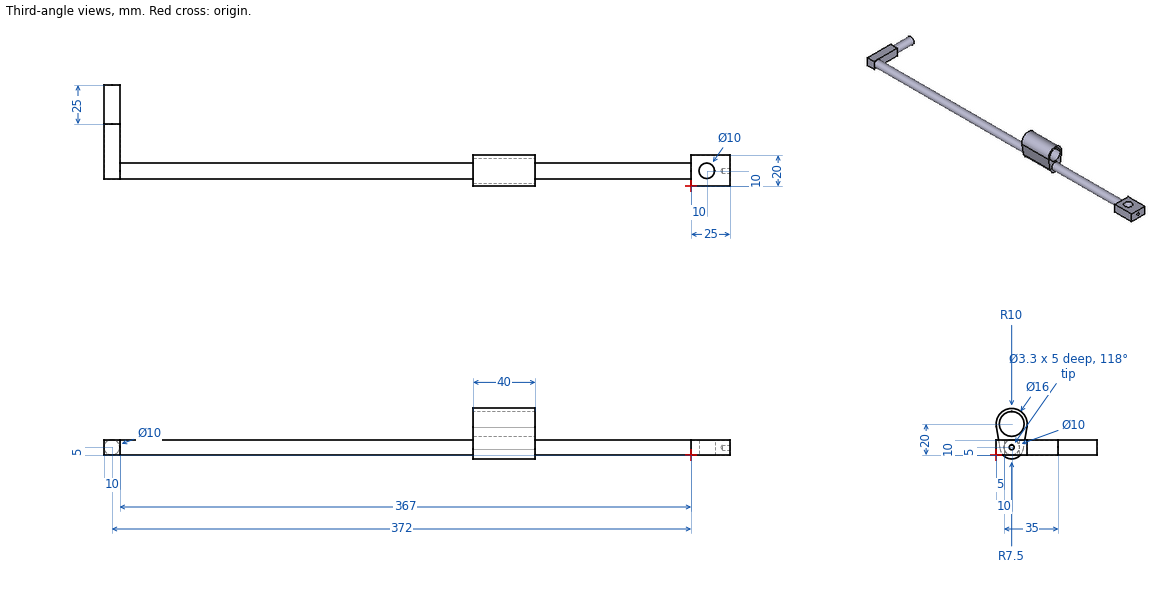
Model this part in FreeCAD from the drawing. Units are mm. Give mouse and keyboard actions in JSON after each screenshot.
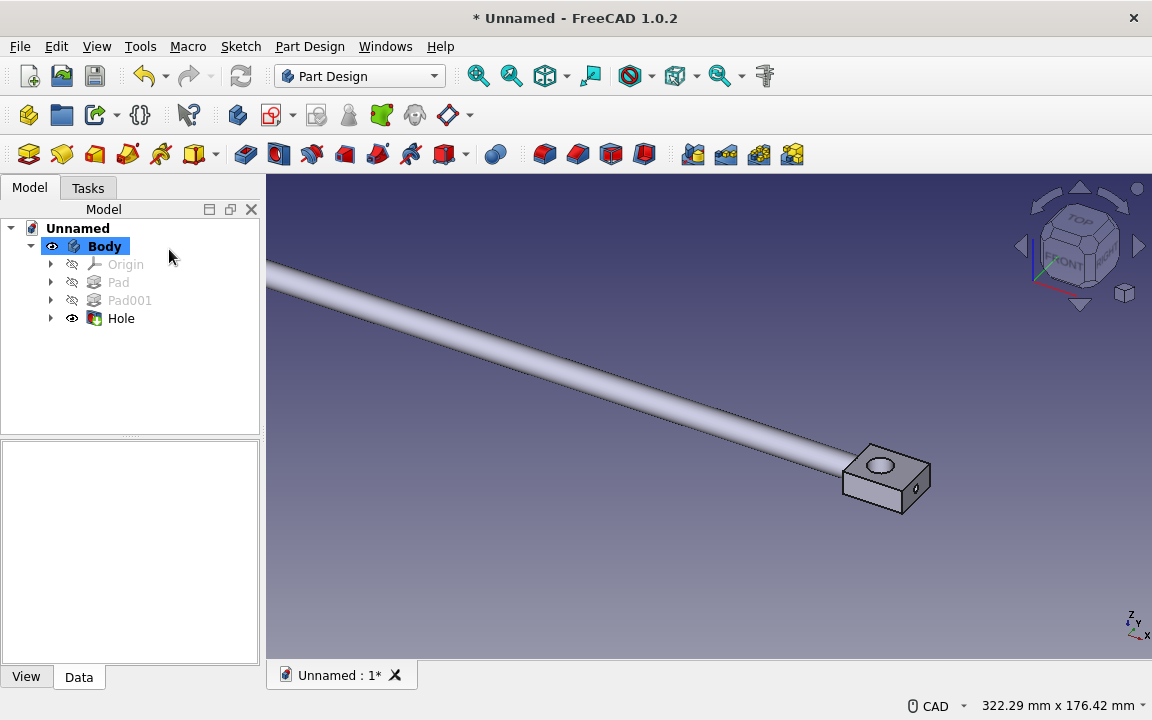
{"action": "key", "text": "v f"}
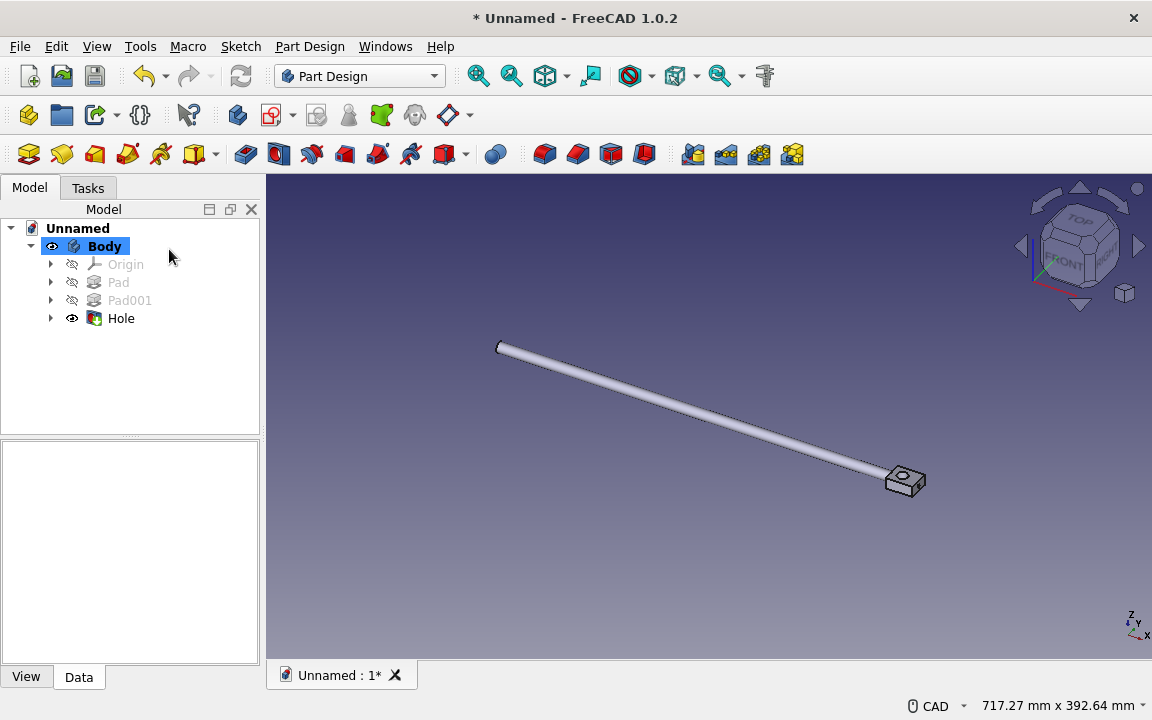
{"action": "key", "text": "6"}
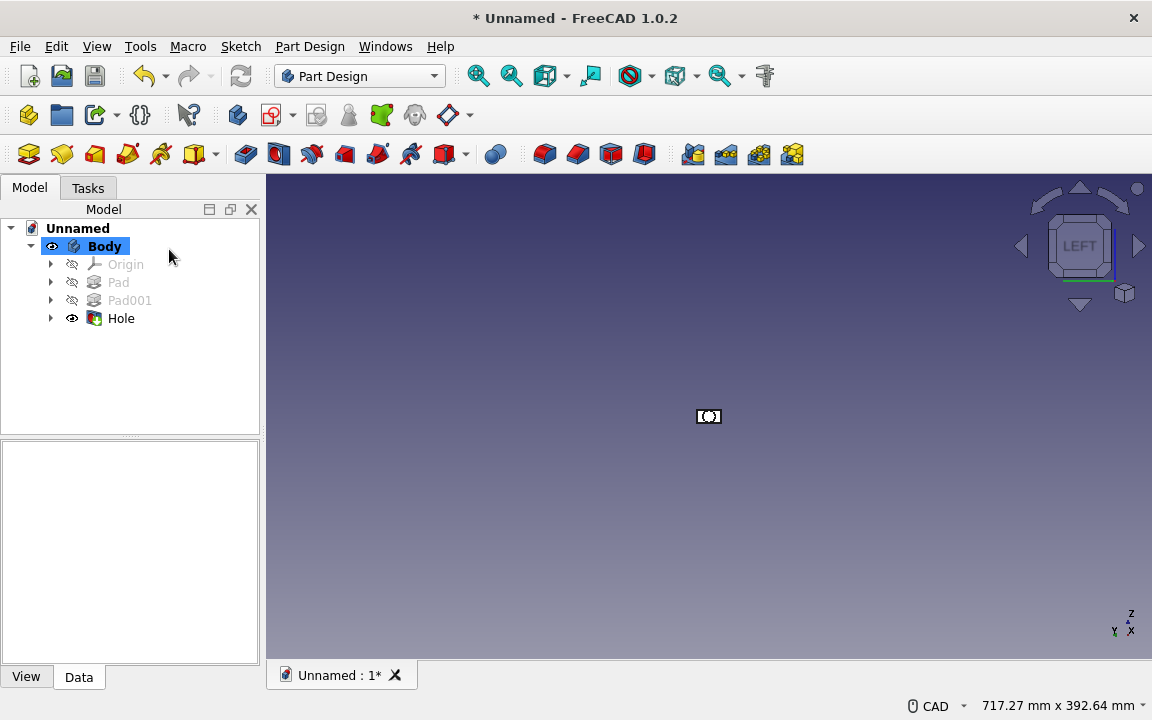
{"action": "left_click", "coordinate": [479, 76]}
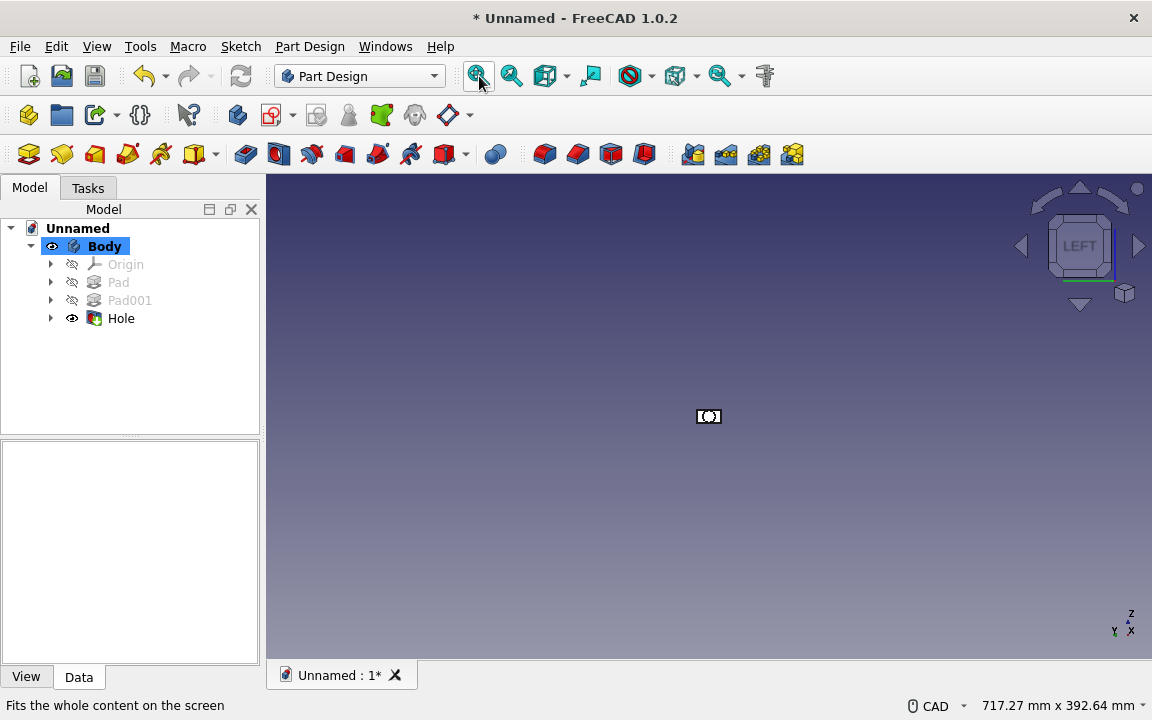
{"action": "scroll", "coordinate": [709, 415], "scroll_direction": "up", "scroll_amount": 4}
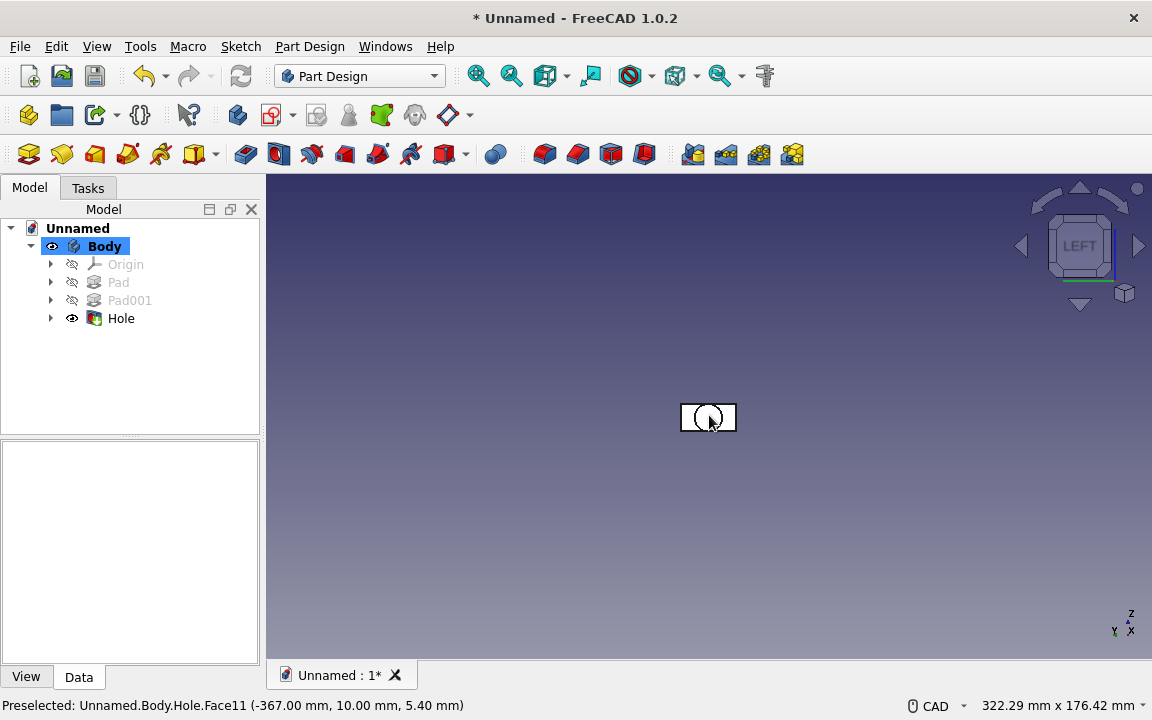
{"action": "left_click", "coordinate": [708, 417]}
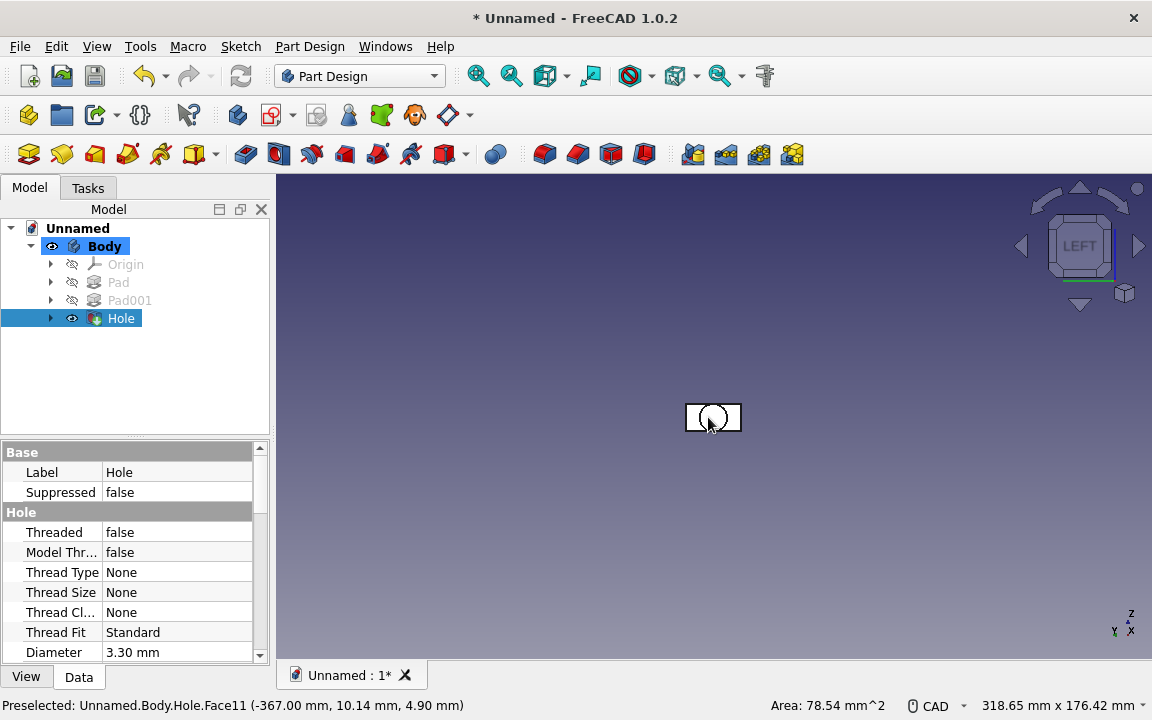
{"action": "left_click", "coordinate": [270, 116]}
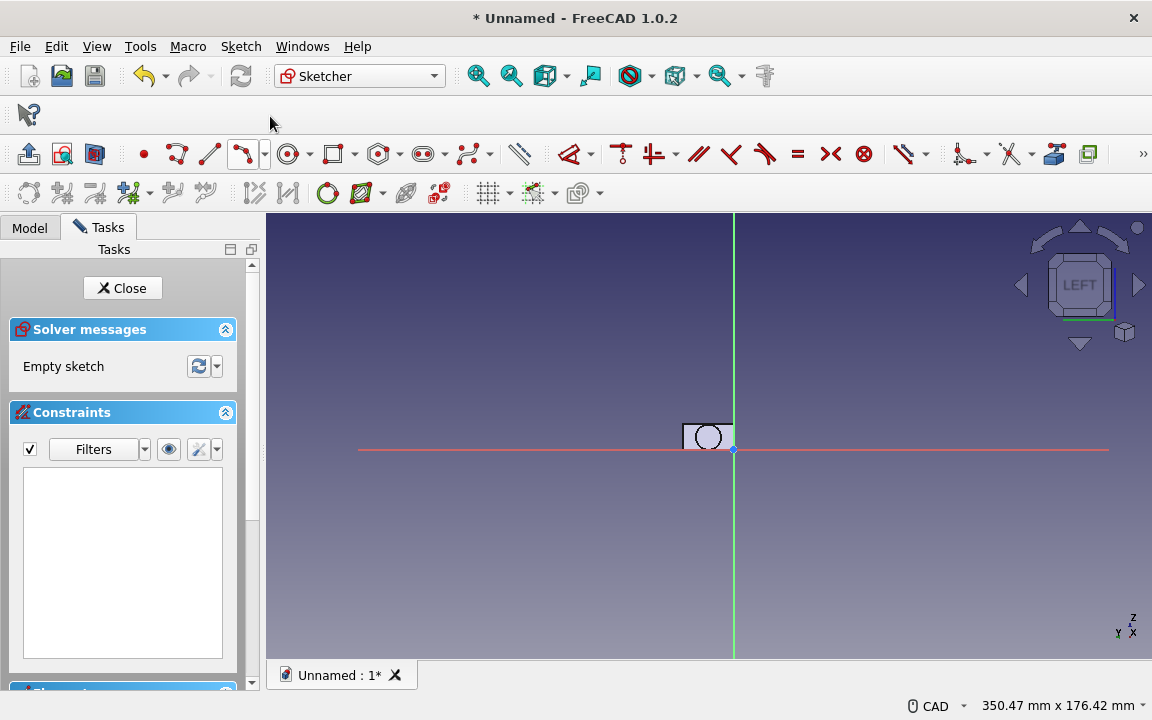
{"action": "scroll", "coordinate": [694, 437], "scroll_direction": "up", "scroll_amount": 8}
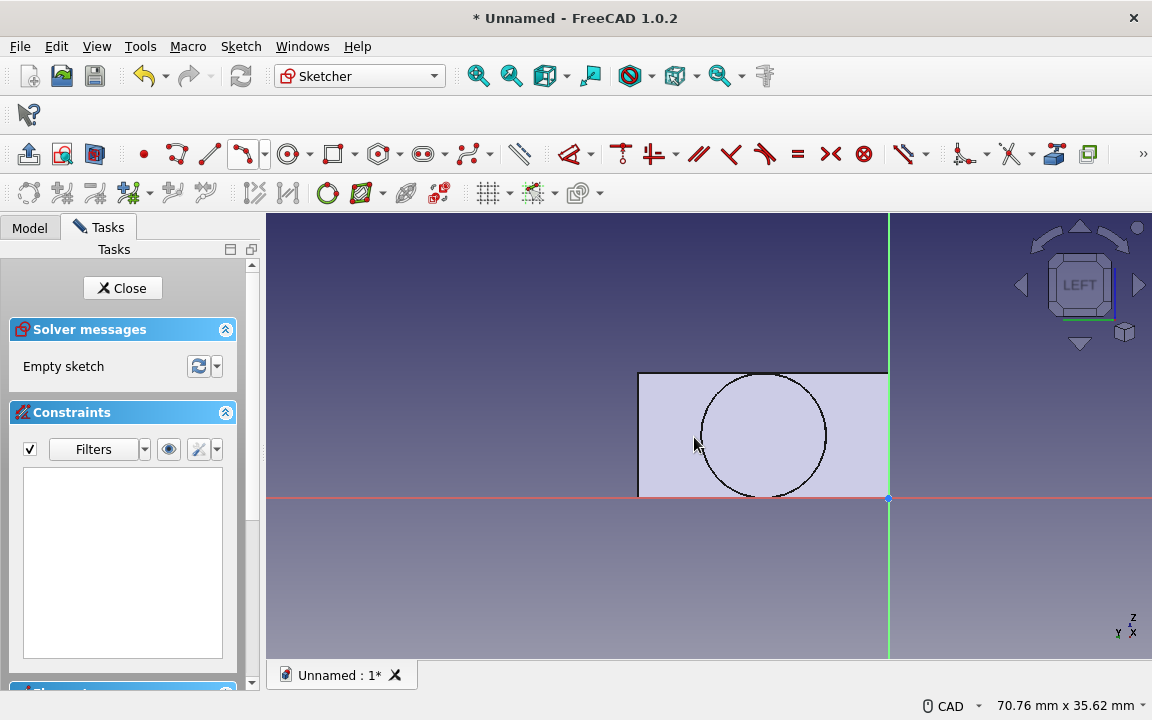
{"action": "key", "text": "g r"}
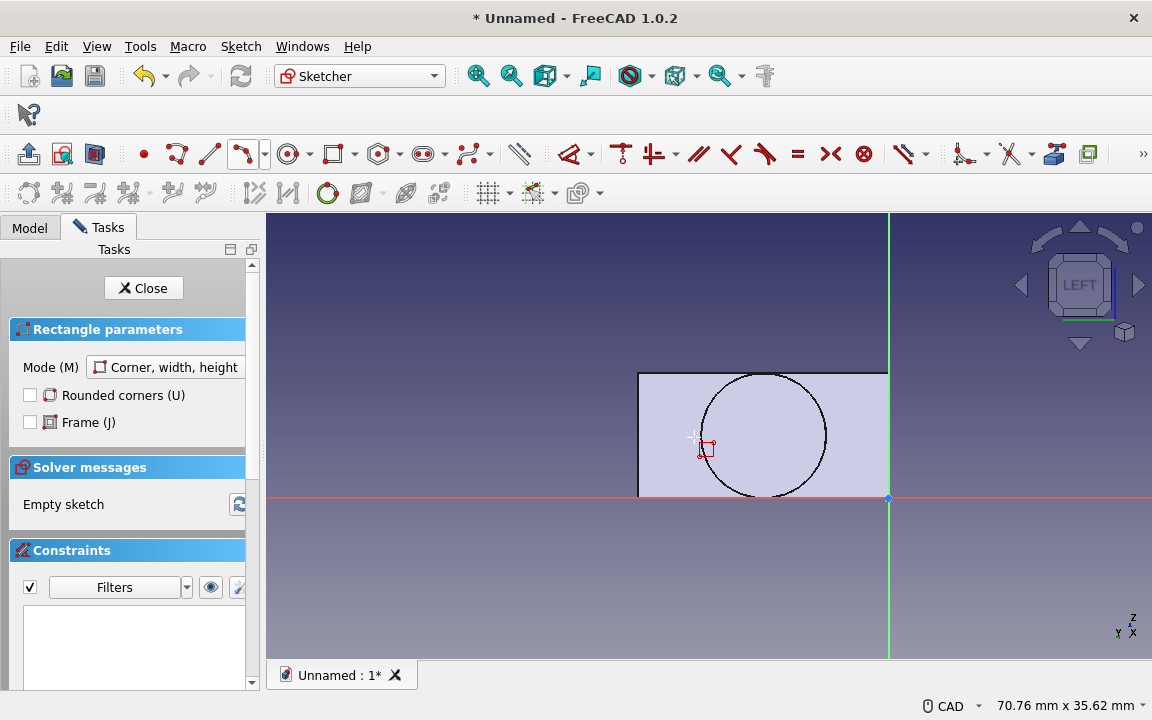
{"action": "left_click", "coordinate": [388, 373]}
{"action": "left_click", "coordinate": [826, 498]}
{"action": "key", "text": "Escape"}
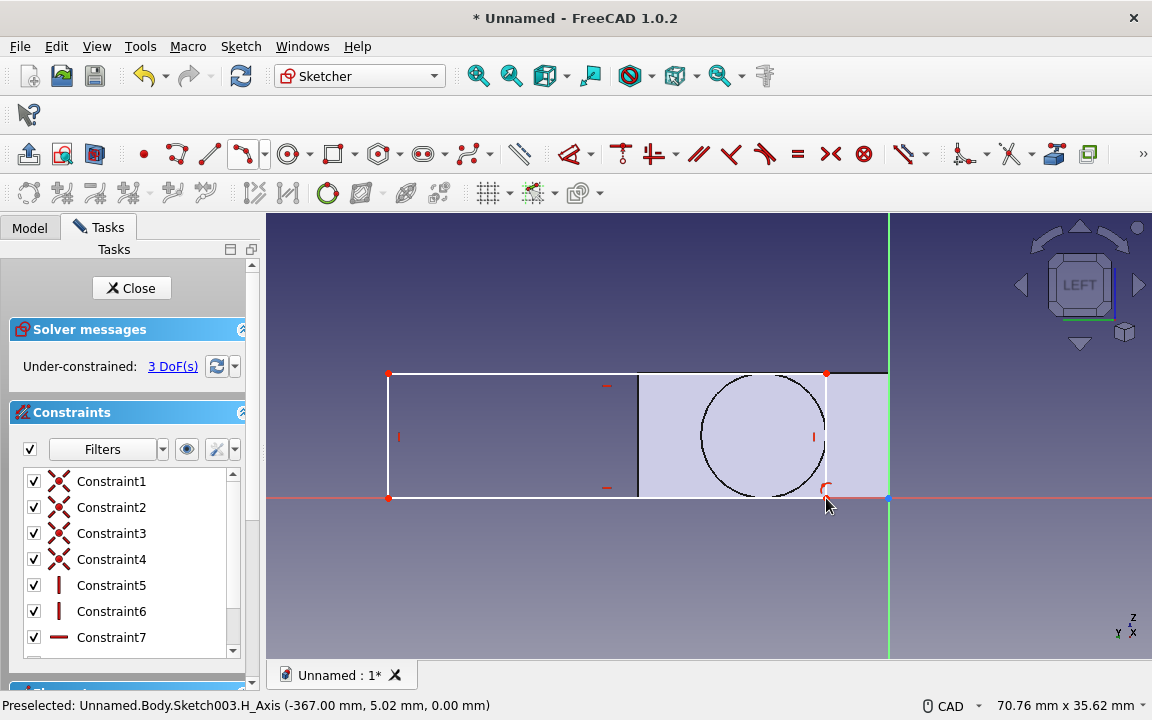
{"action": "key", "text": "d"}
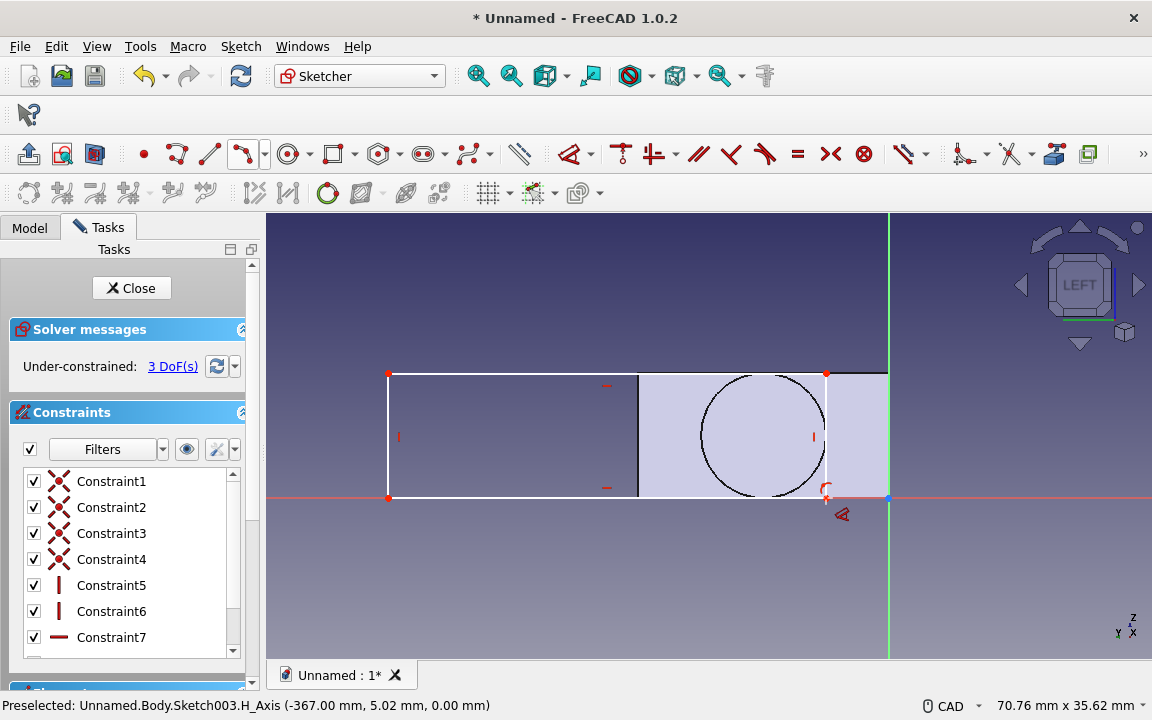
{"action": "left_click", "coordinate": [388, 411]}
{"action": "left_click", "coordinate": [354, 436]}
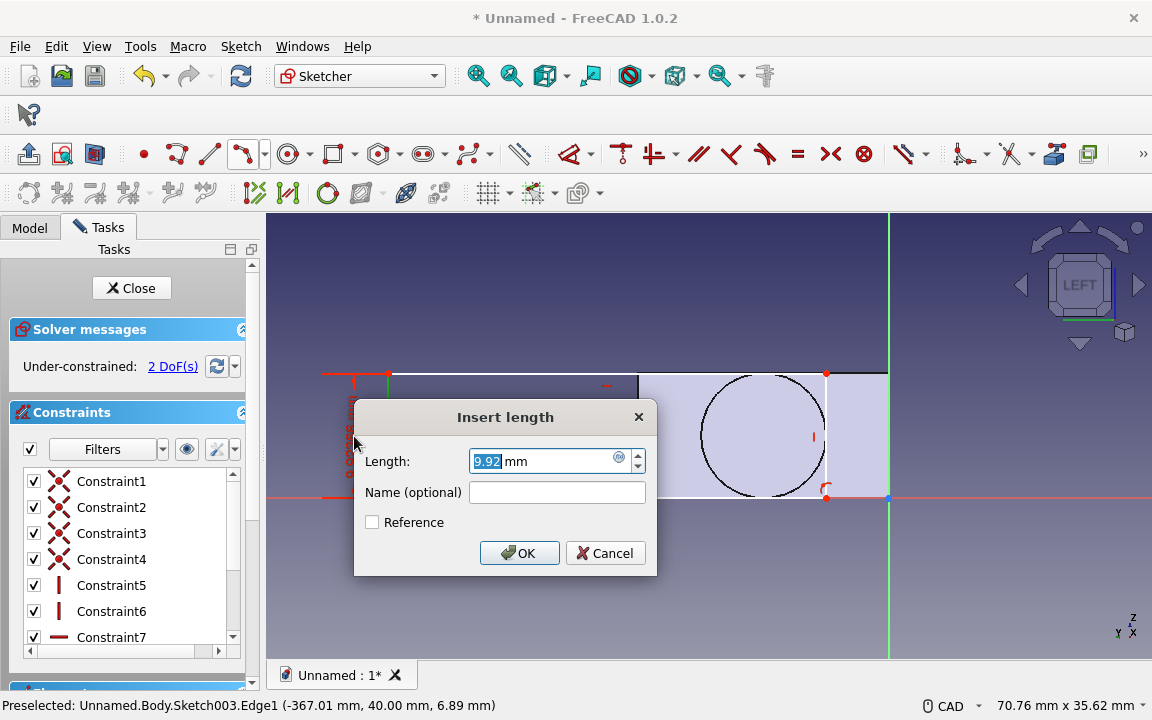
{"action": "type", "text": "10"}
{"action": "key", "text": "Return"}